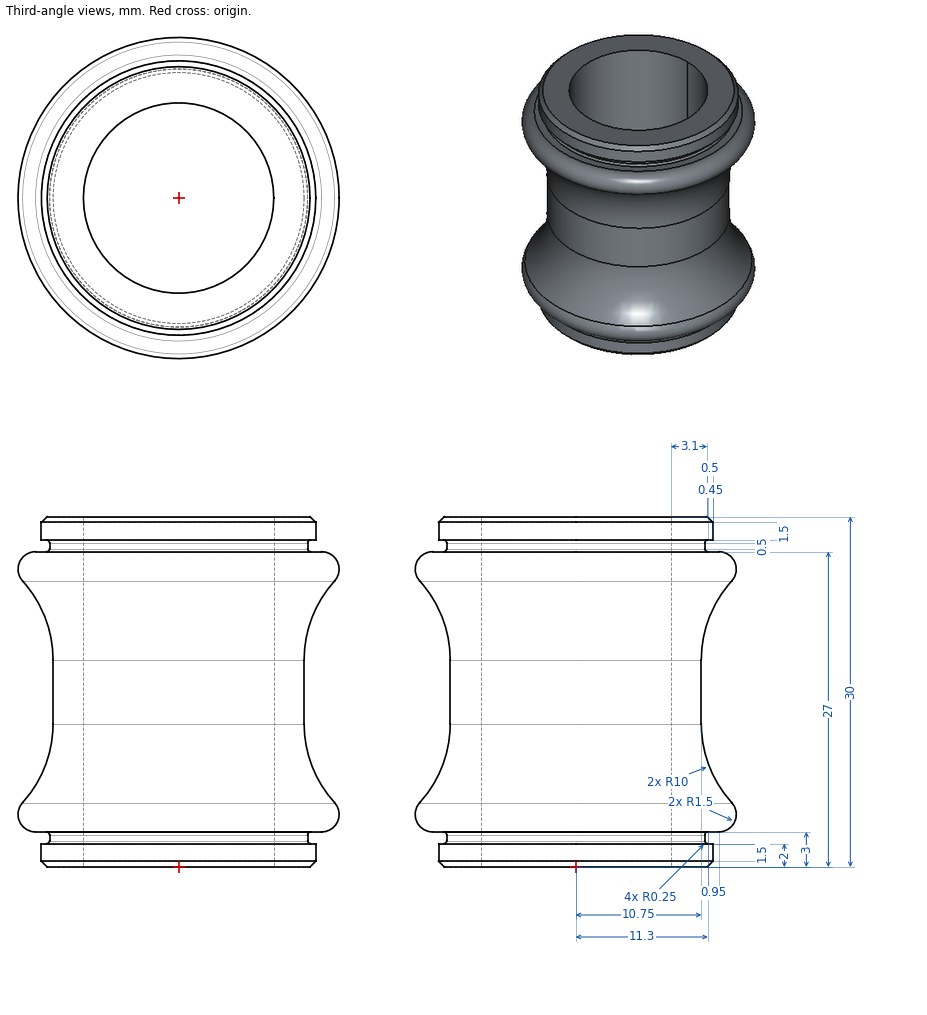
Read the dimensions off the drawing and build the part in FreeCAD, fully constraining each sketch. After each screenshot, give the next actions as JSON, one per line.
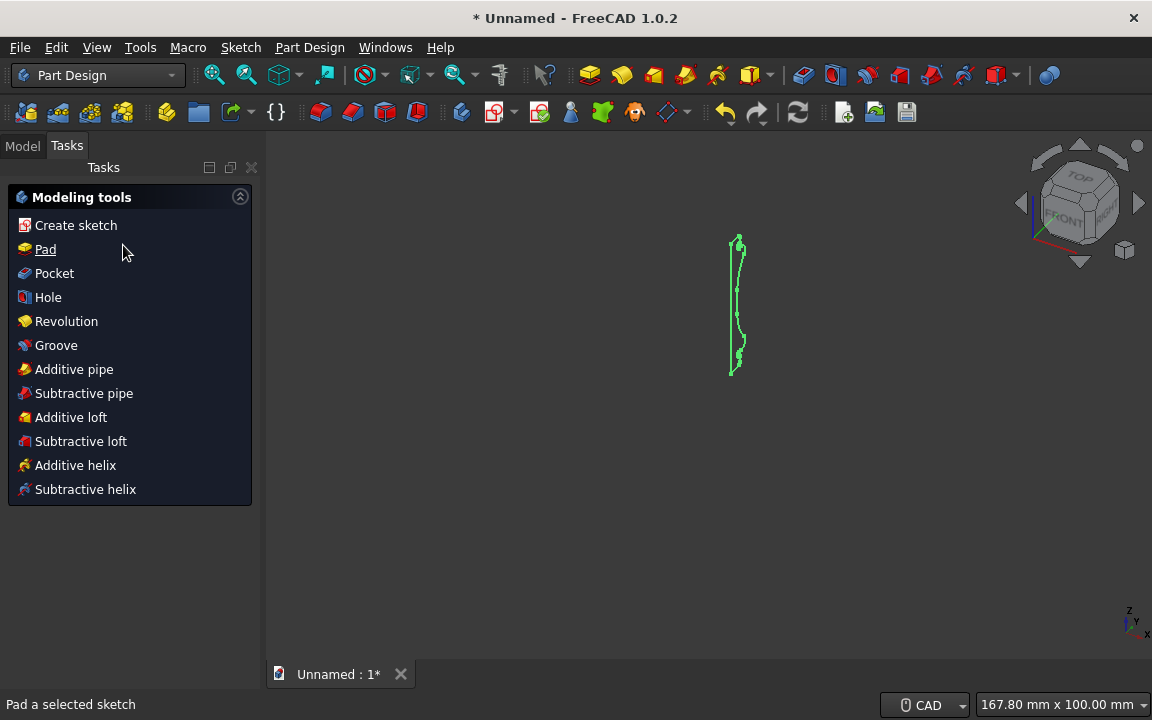
{"action": "left_click", "coordinate": [622, 76]}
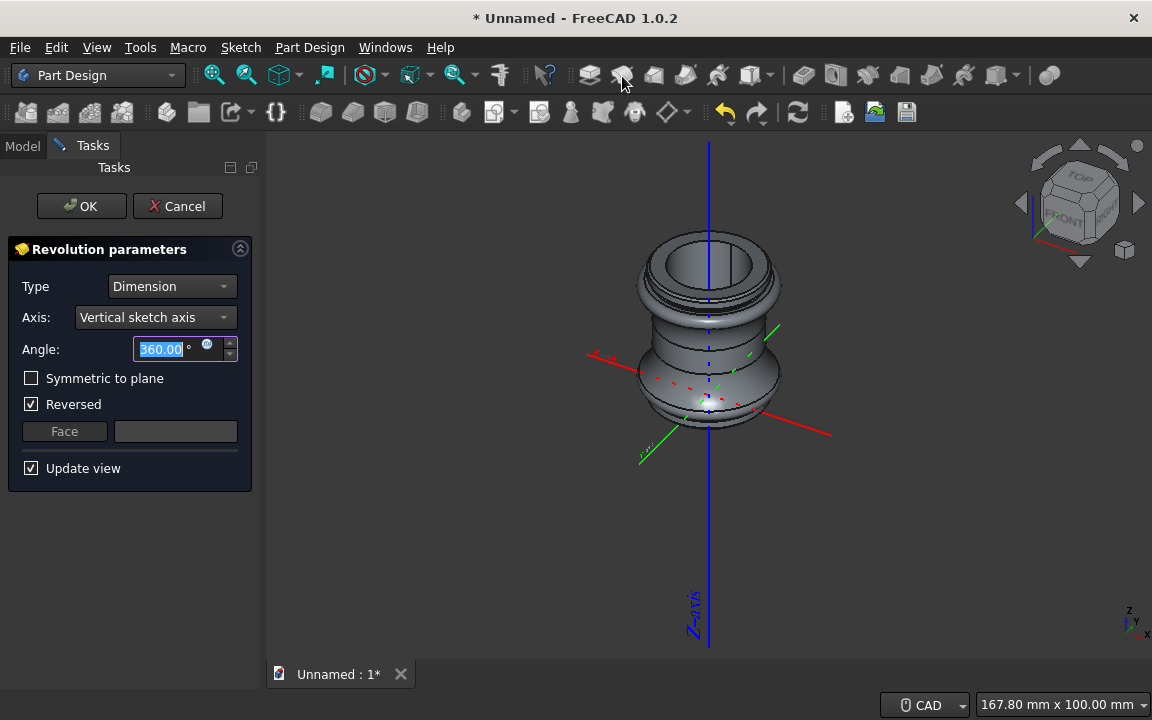
{"action": "left_click", "coordinate": [82, 206]}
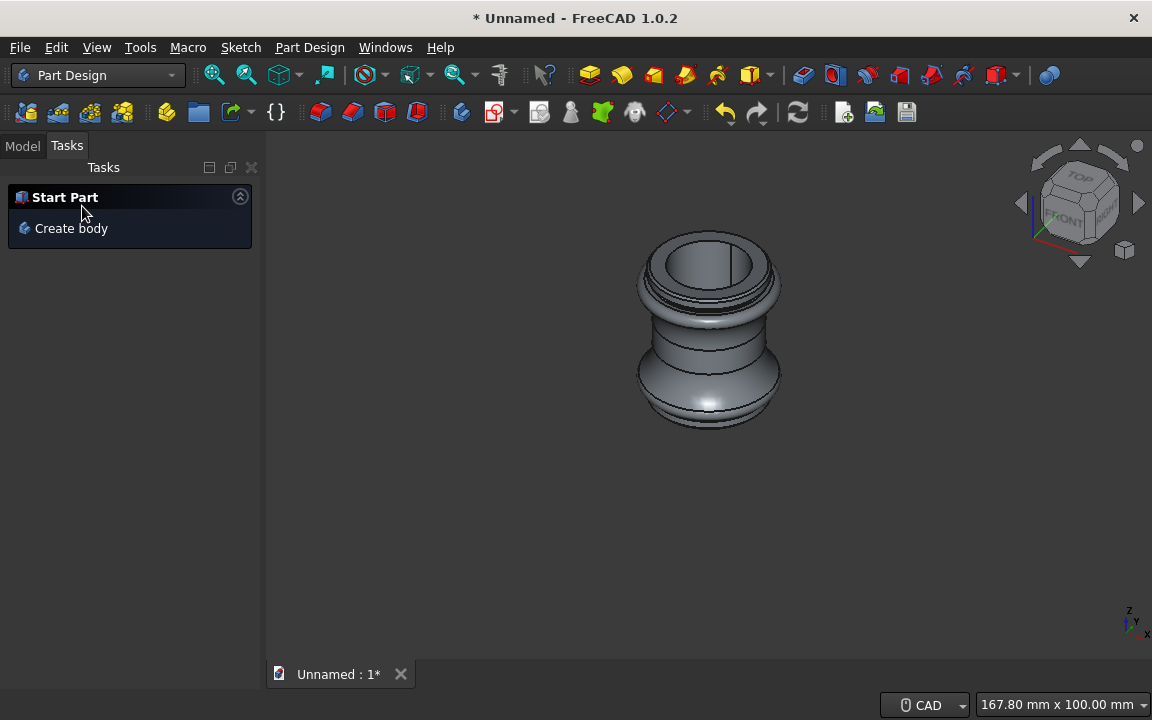
{"action": "key", "text": "0"}